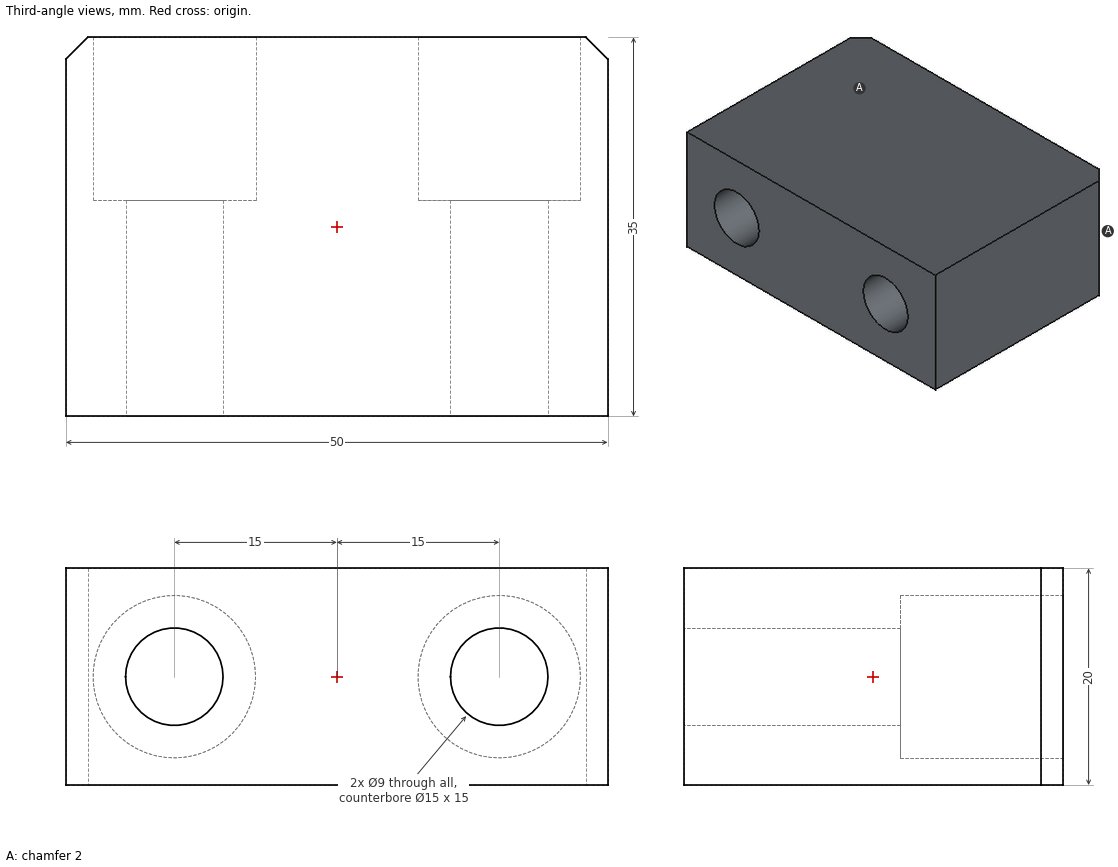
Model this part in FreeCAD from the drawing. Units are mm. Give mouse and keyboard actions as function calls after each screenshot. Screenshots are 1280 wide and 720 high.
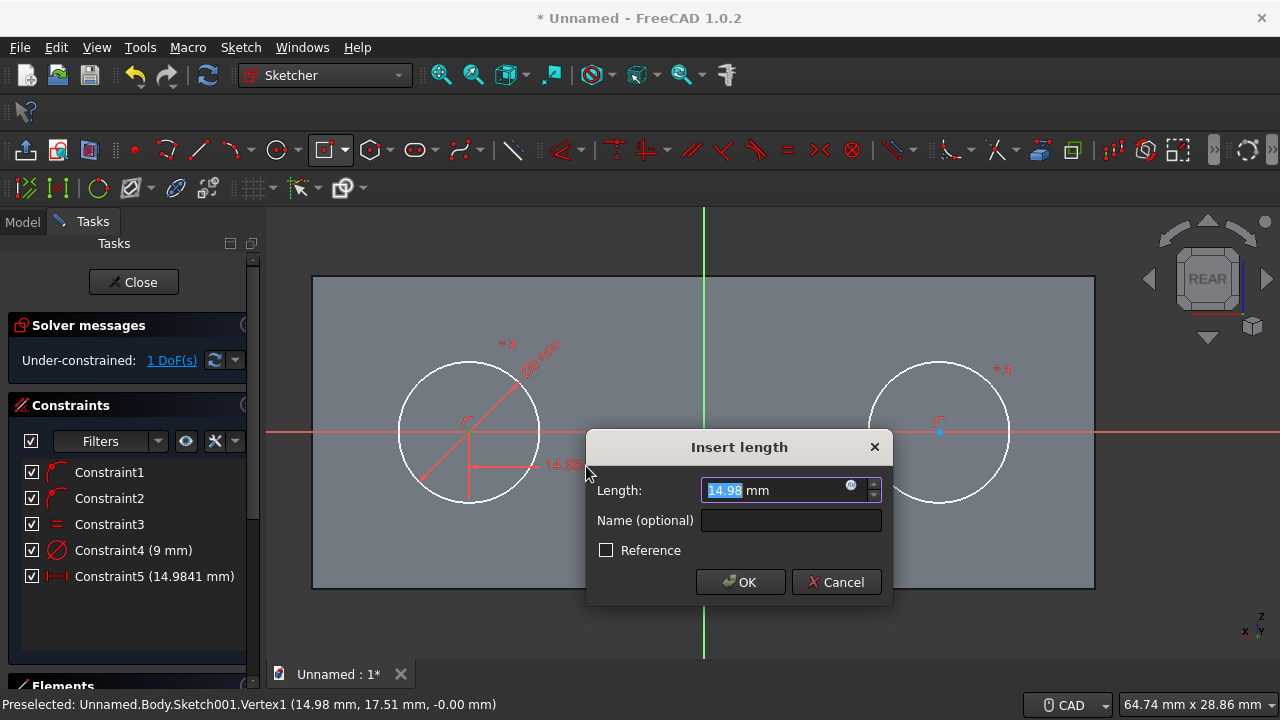
text(15)
key(Return)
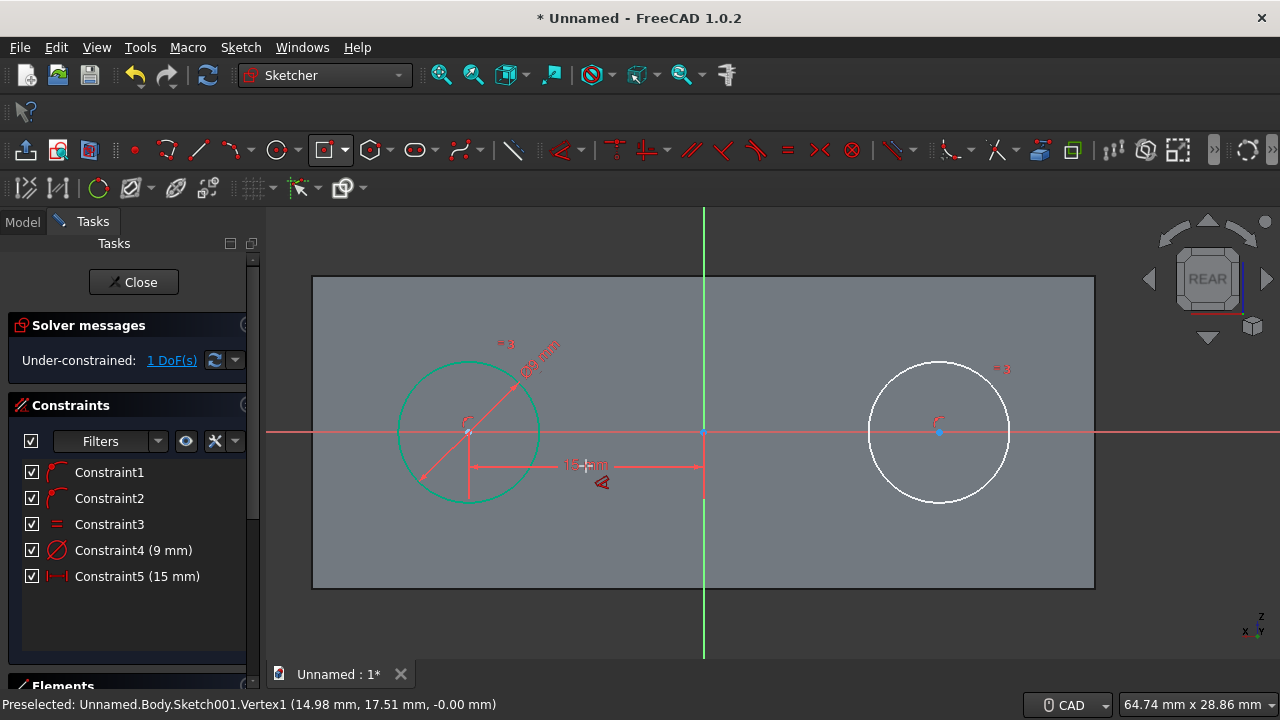
click(939, 432)
click(821, 466)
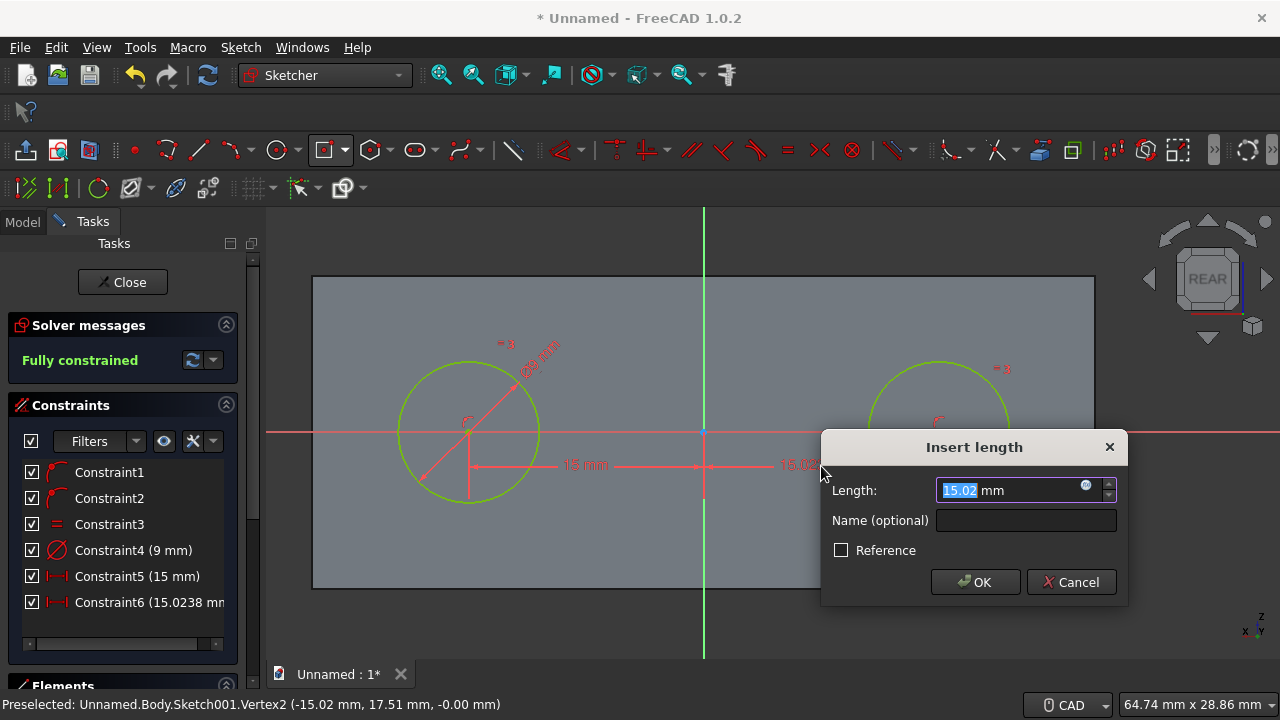
text(15)
key(Return)
key(Escape)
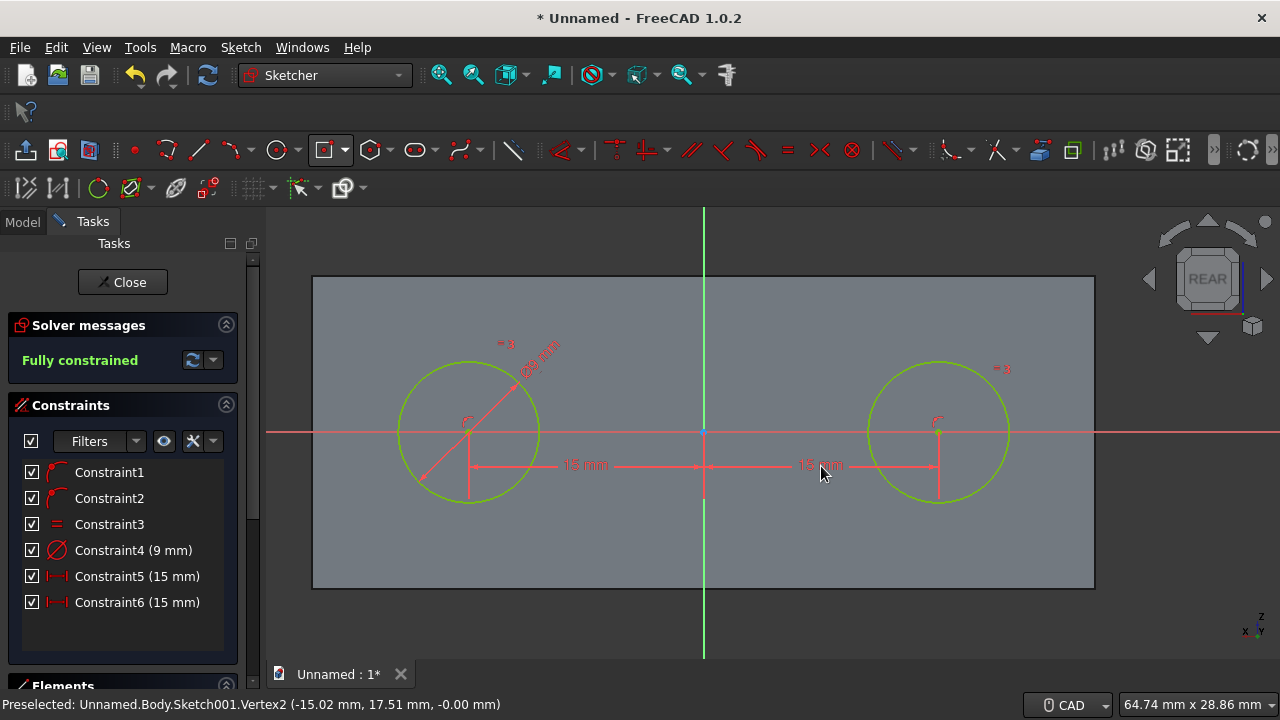
click(123, 282)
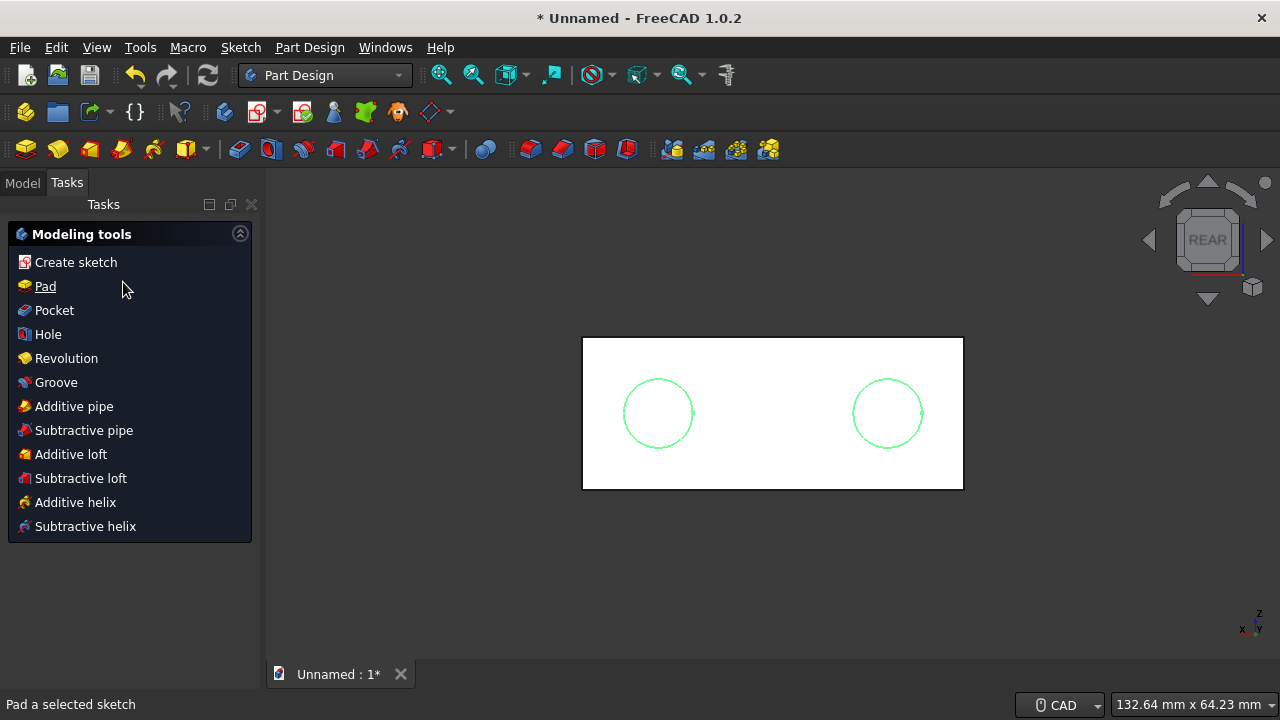
click(272, 150)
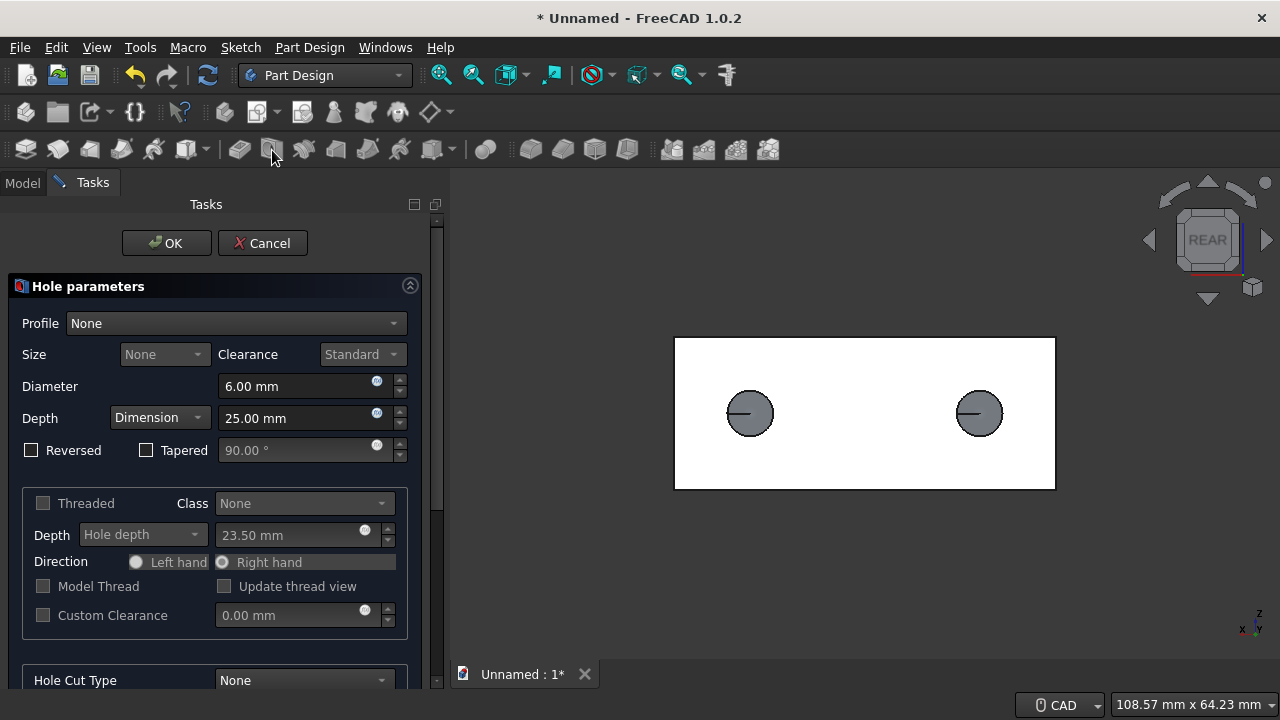
triple_click(305, 386)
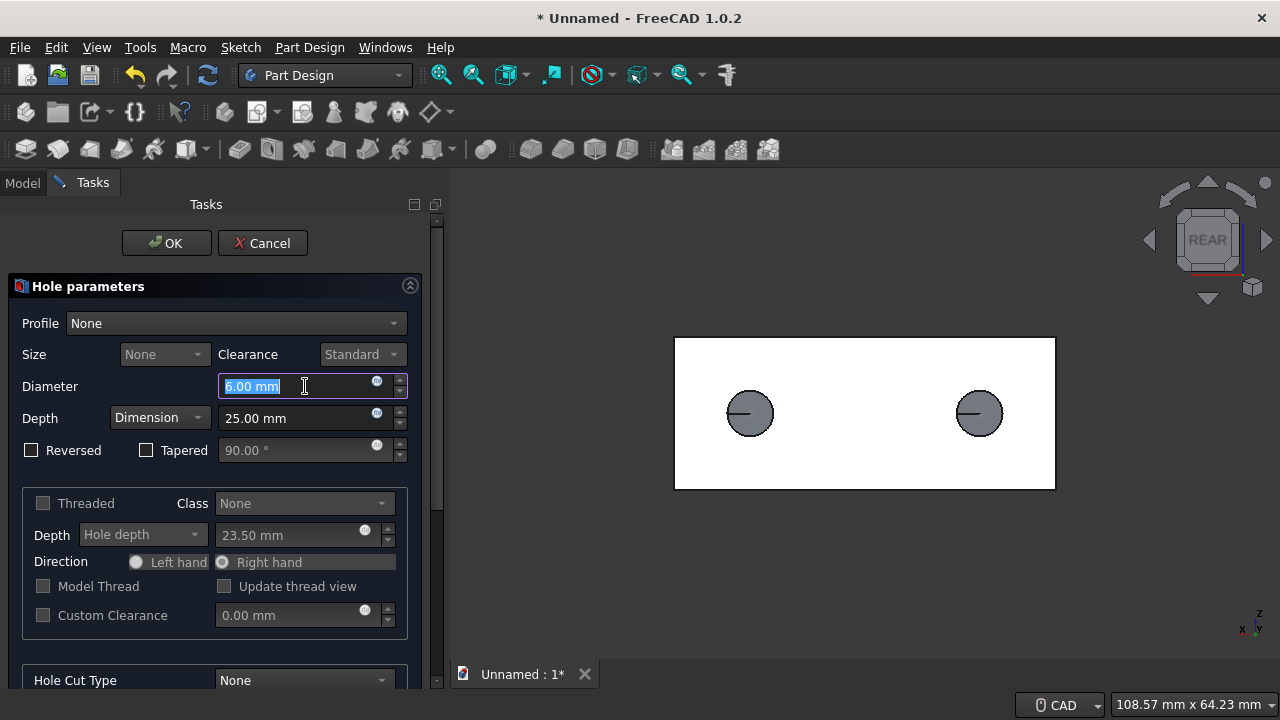
text(9)
key(Tab)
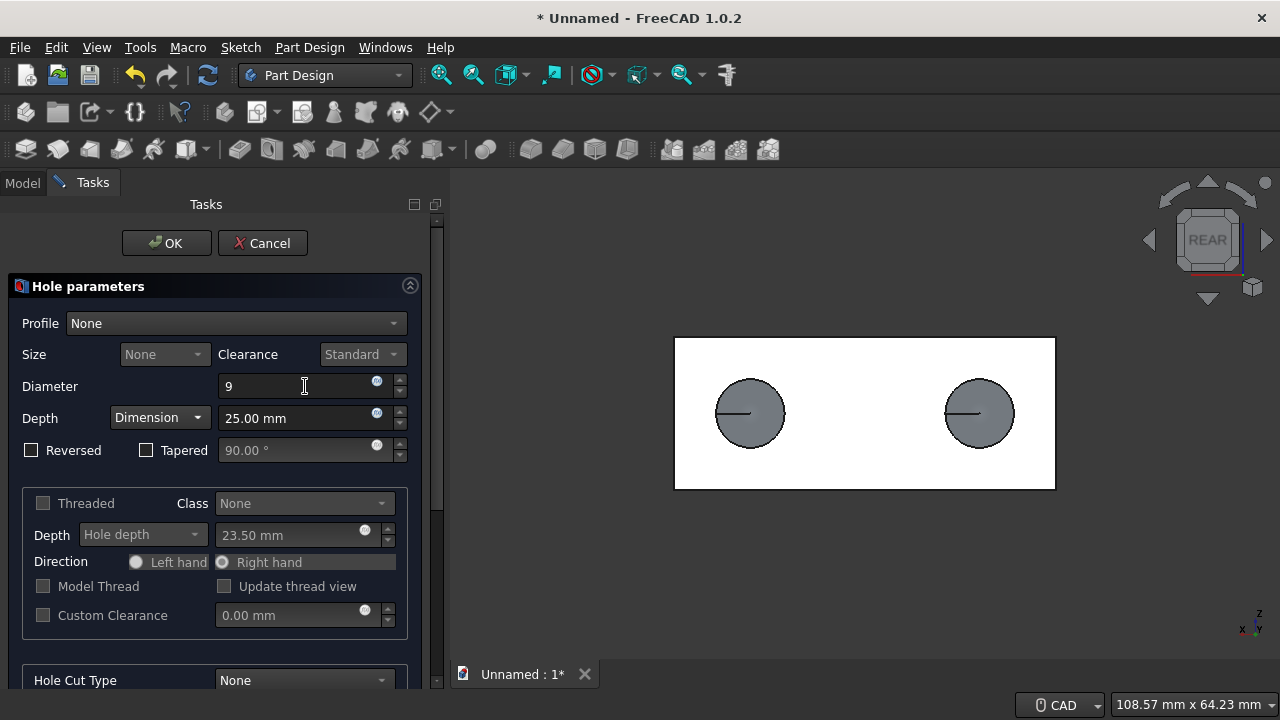
click(161, 418)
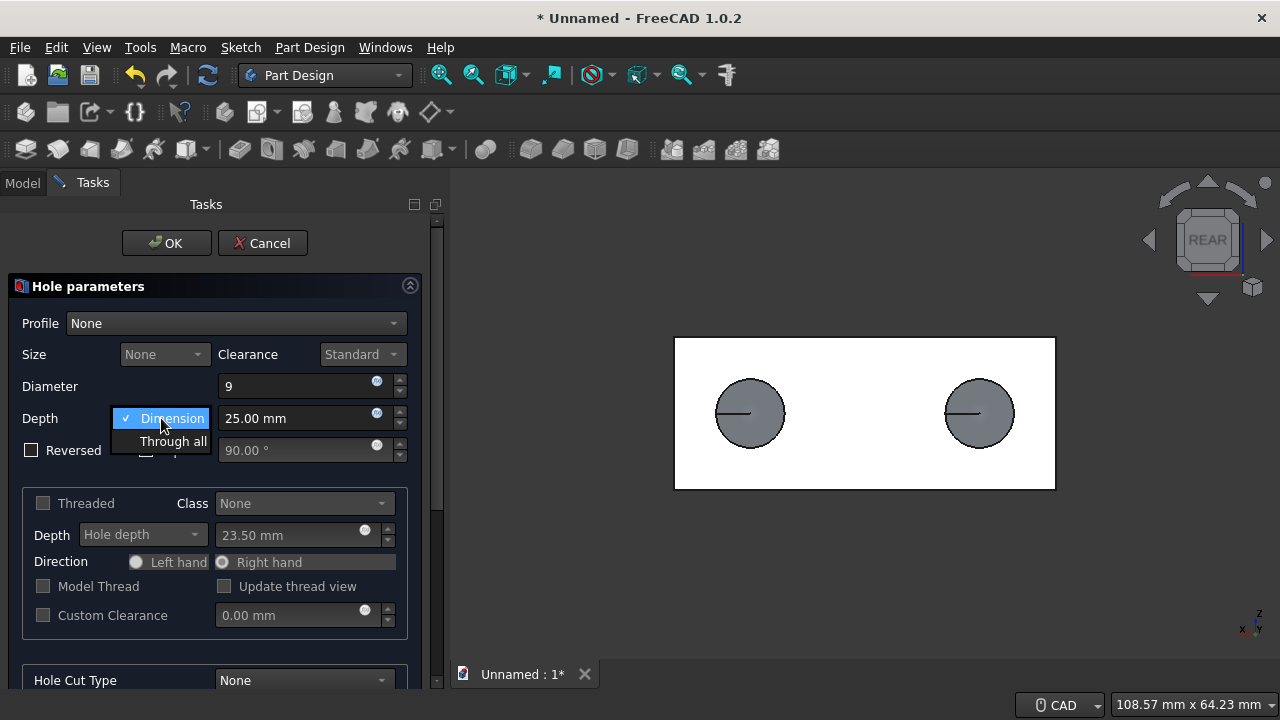
click(160, 442)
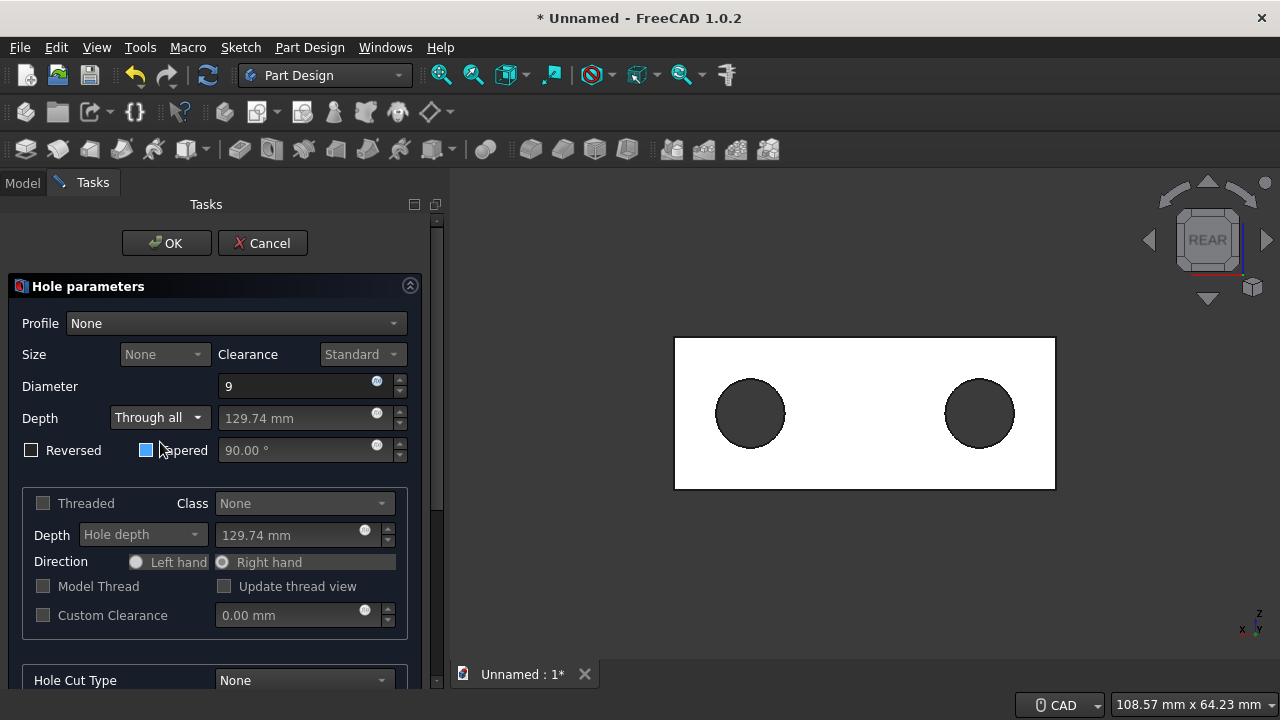
scroll(437, 451, down, 2)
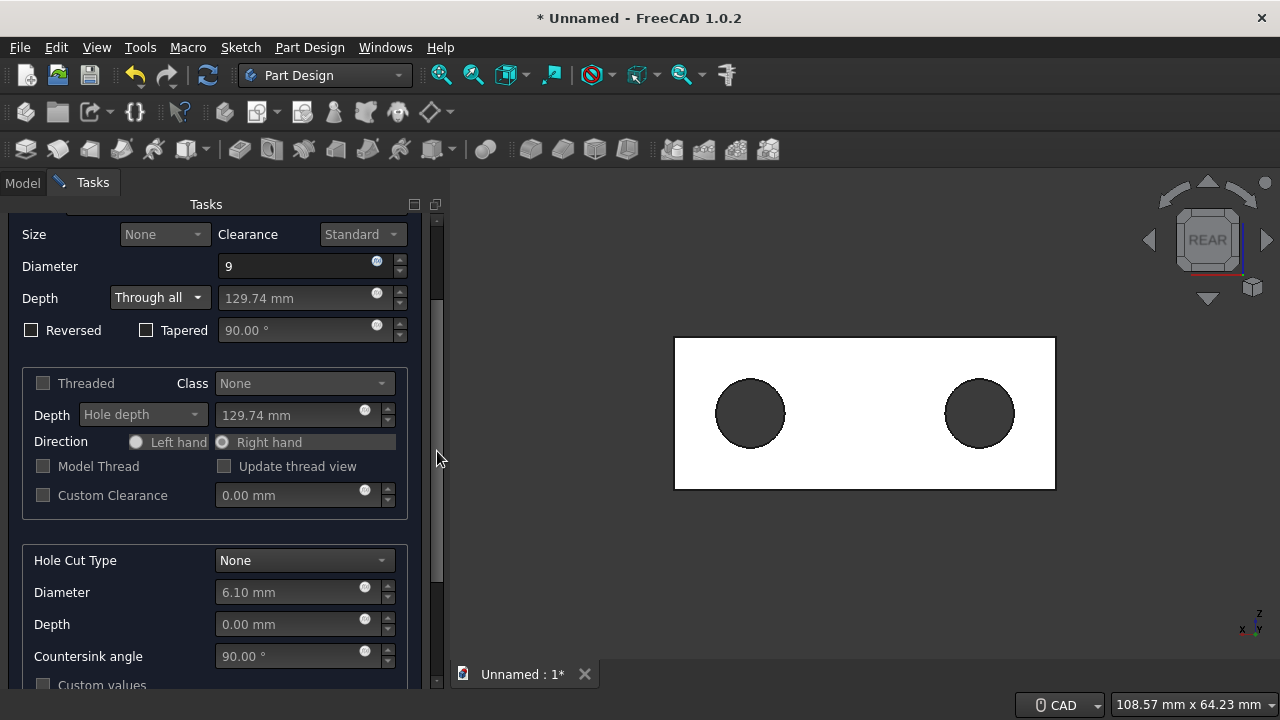
click(306, 560)